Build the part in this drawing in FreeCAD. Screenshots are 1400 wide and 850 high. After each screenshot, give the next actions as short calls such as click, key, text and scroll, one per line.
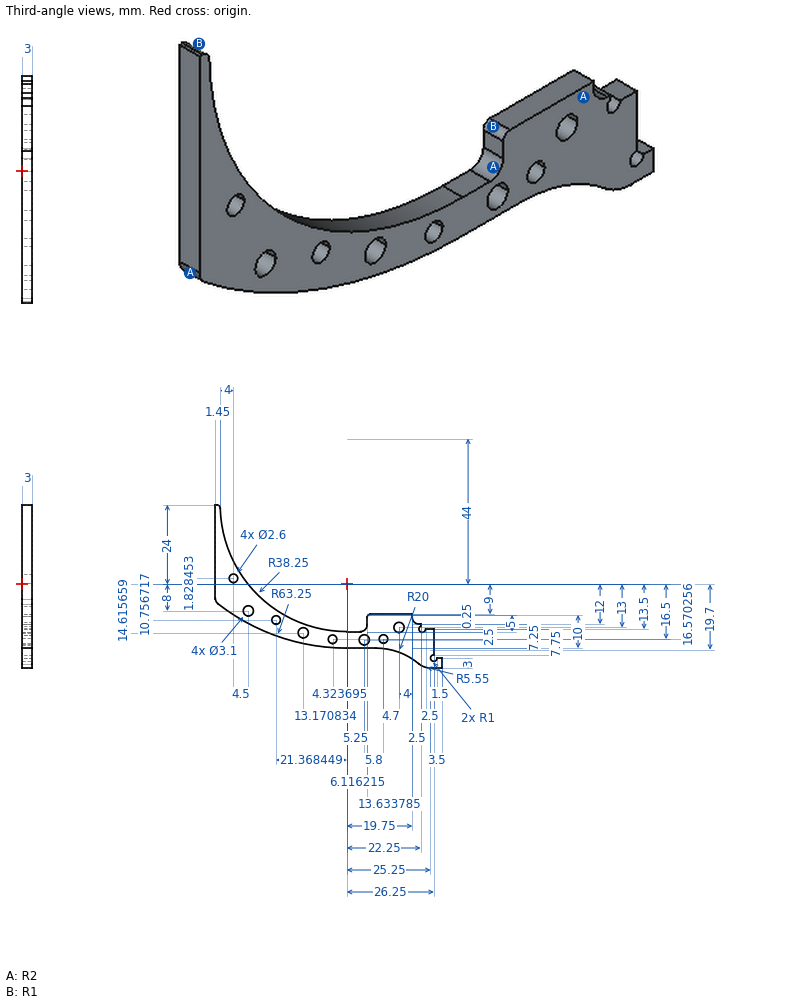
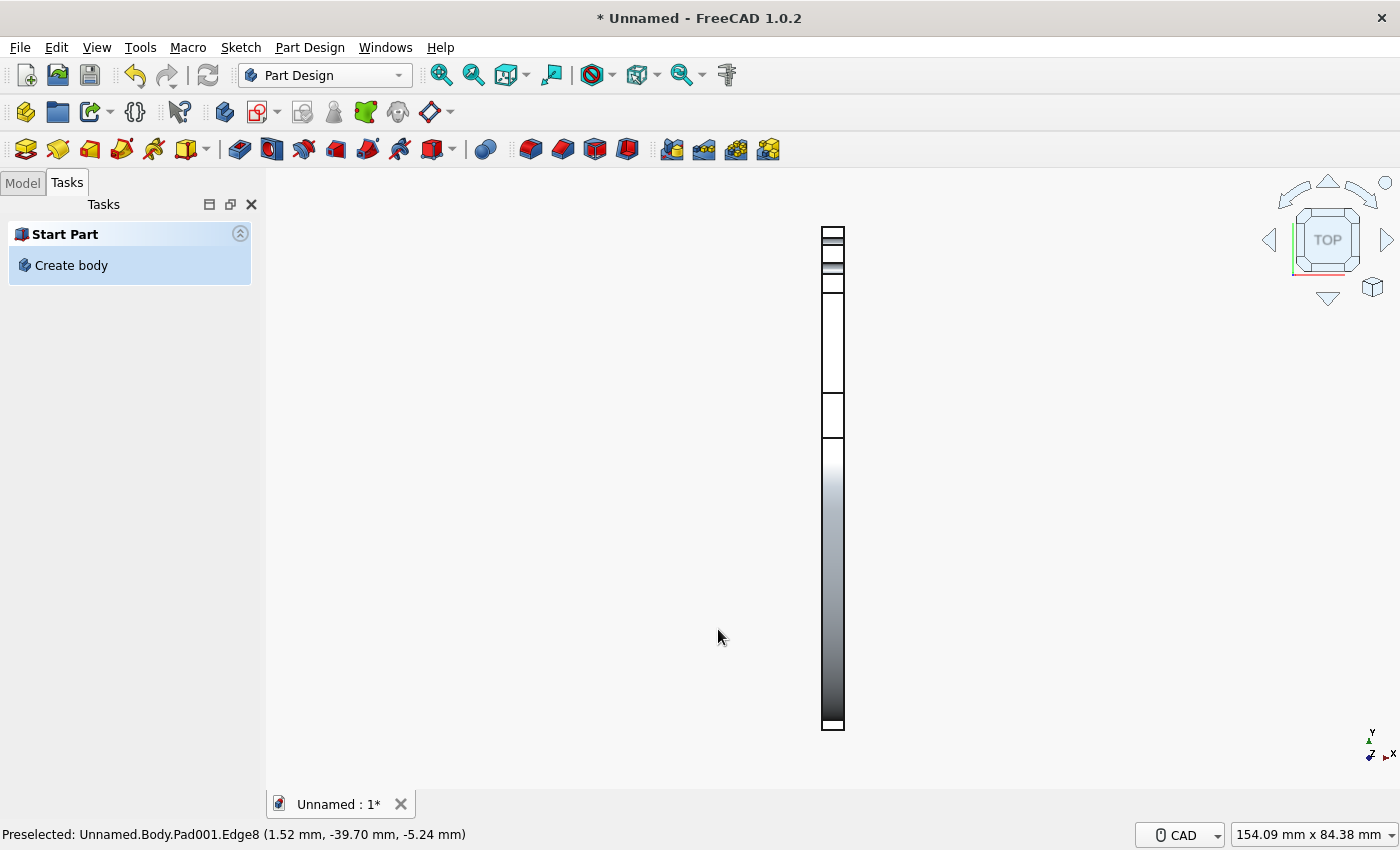
key(1)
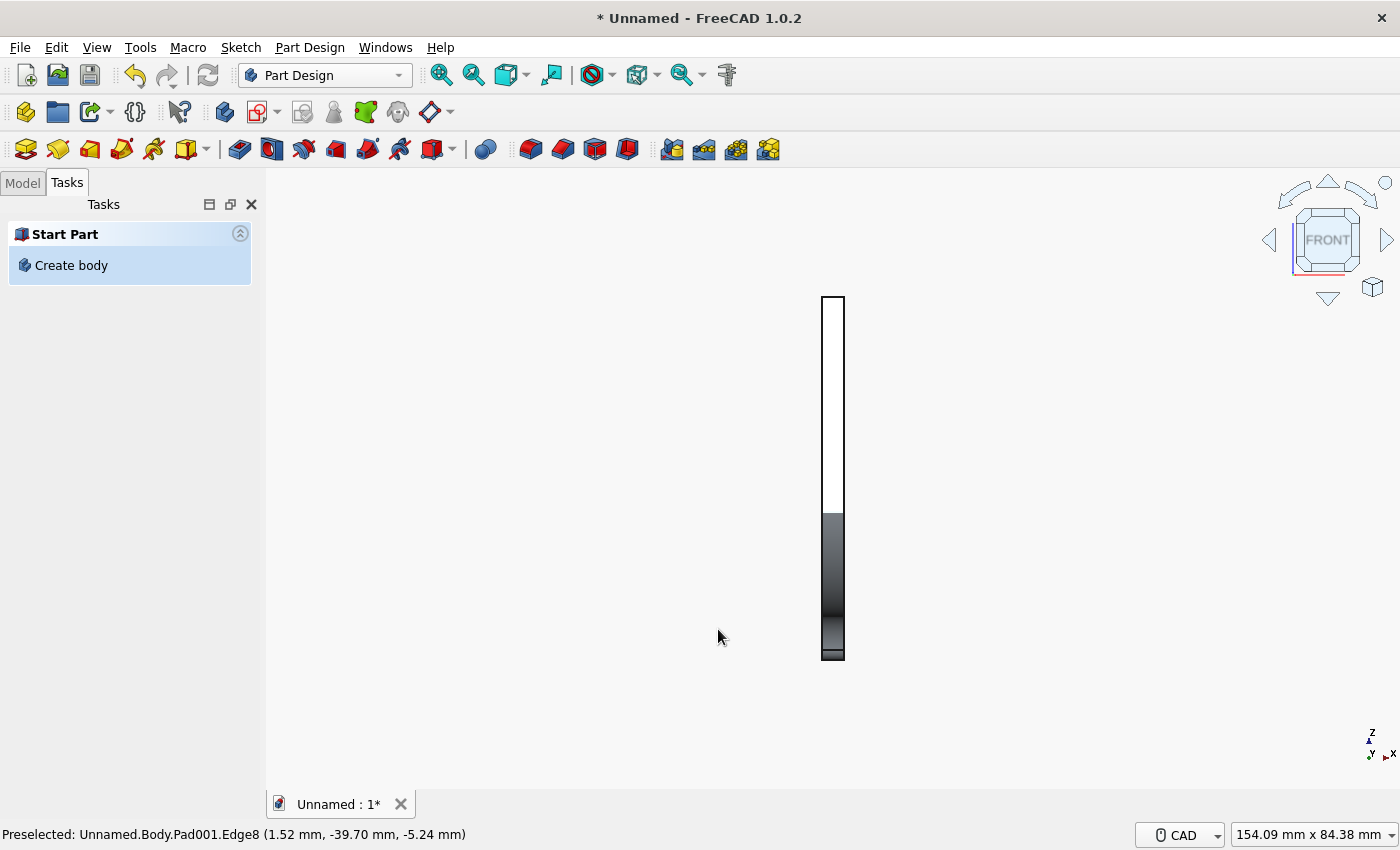
click(833, 511)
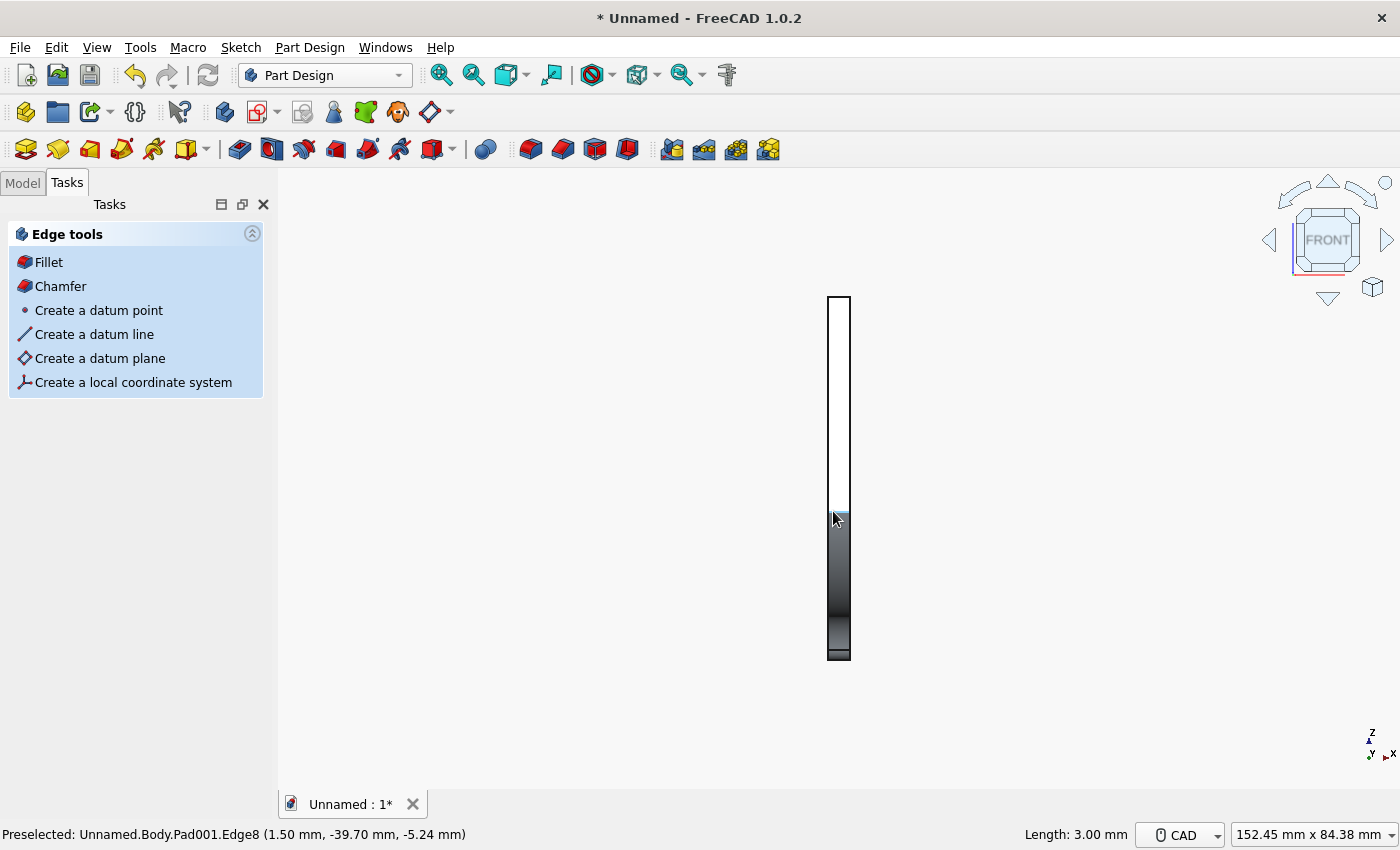
key(3)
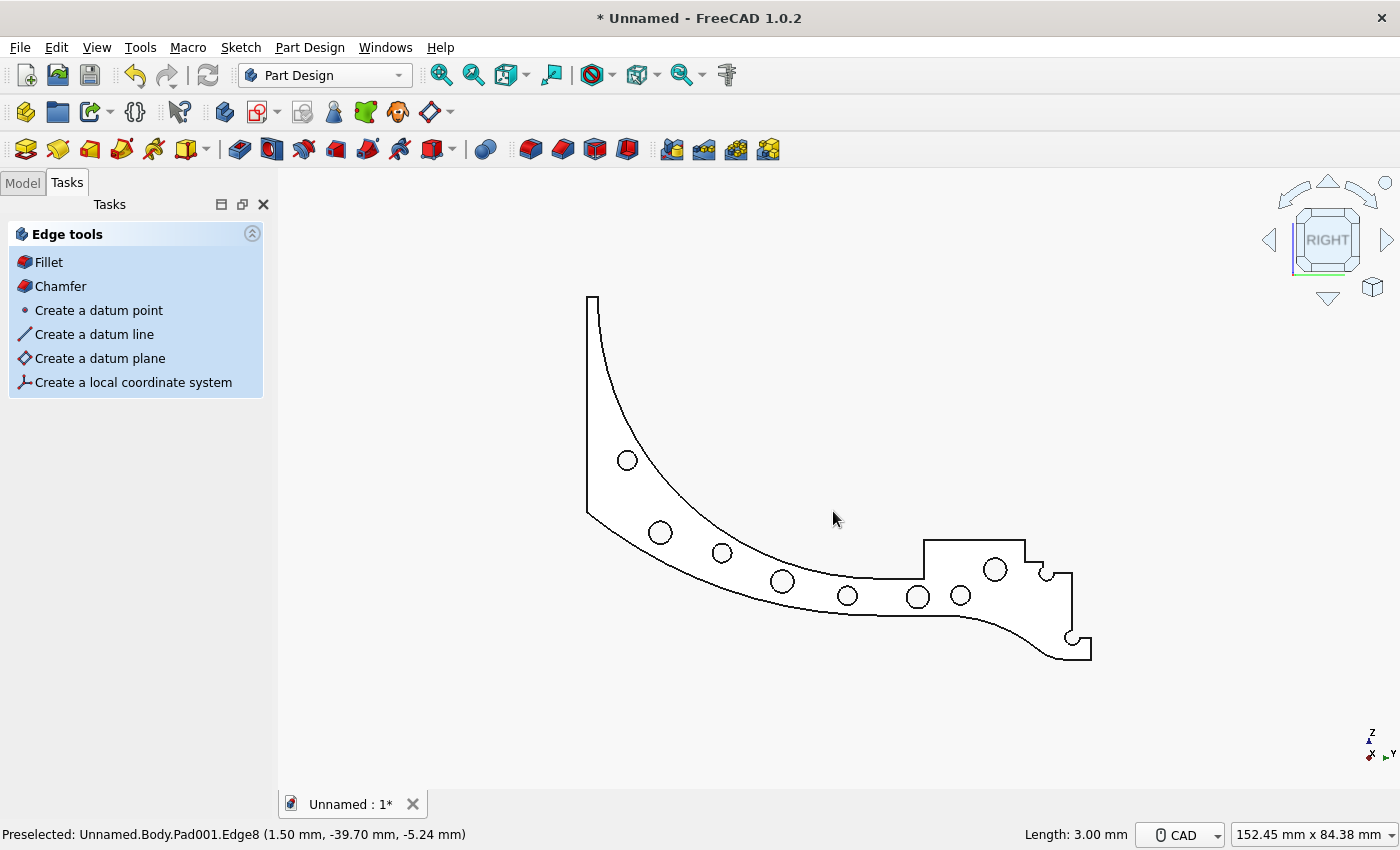
key(5)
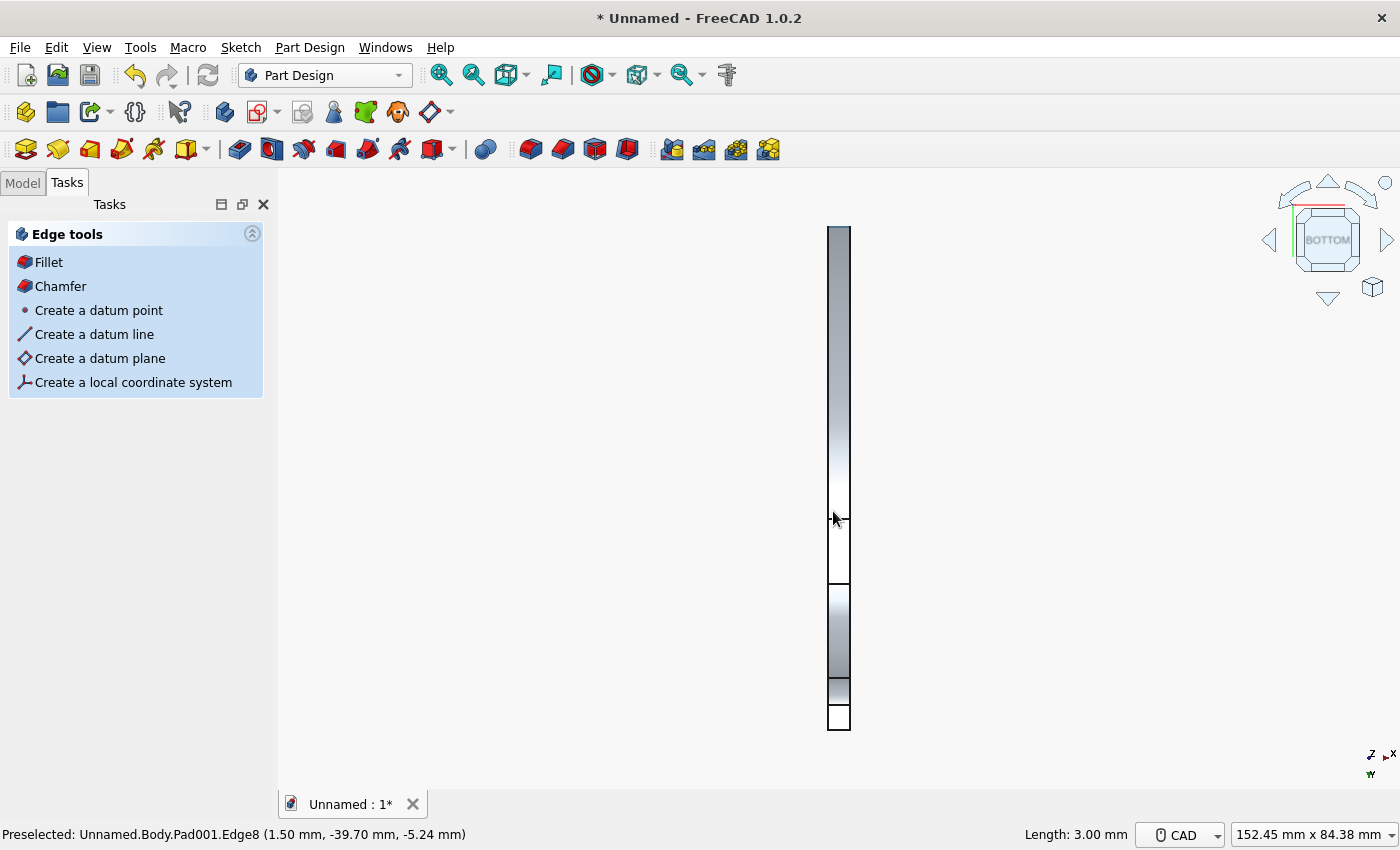
key(4)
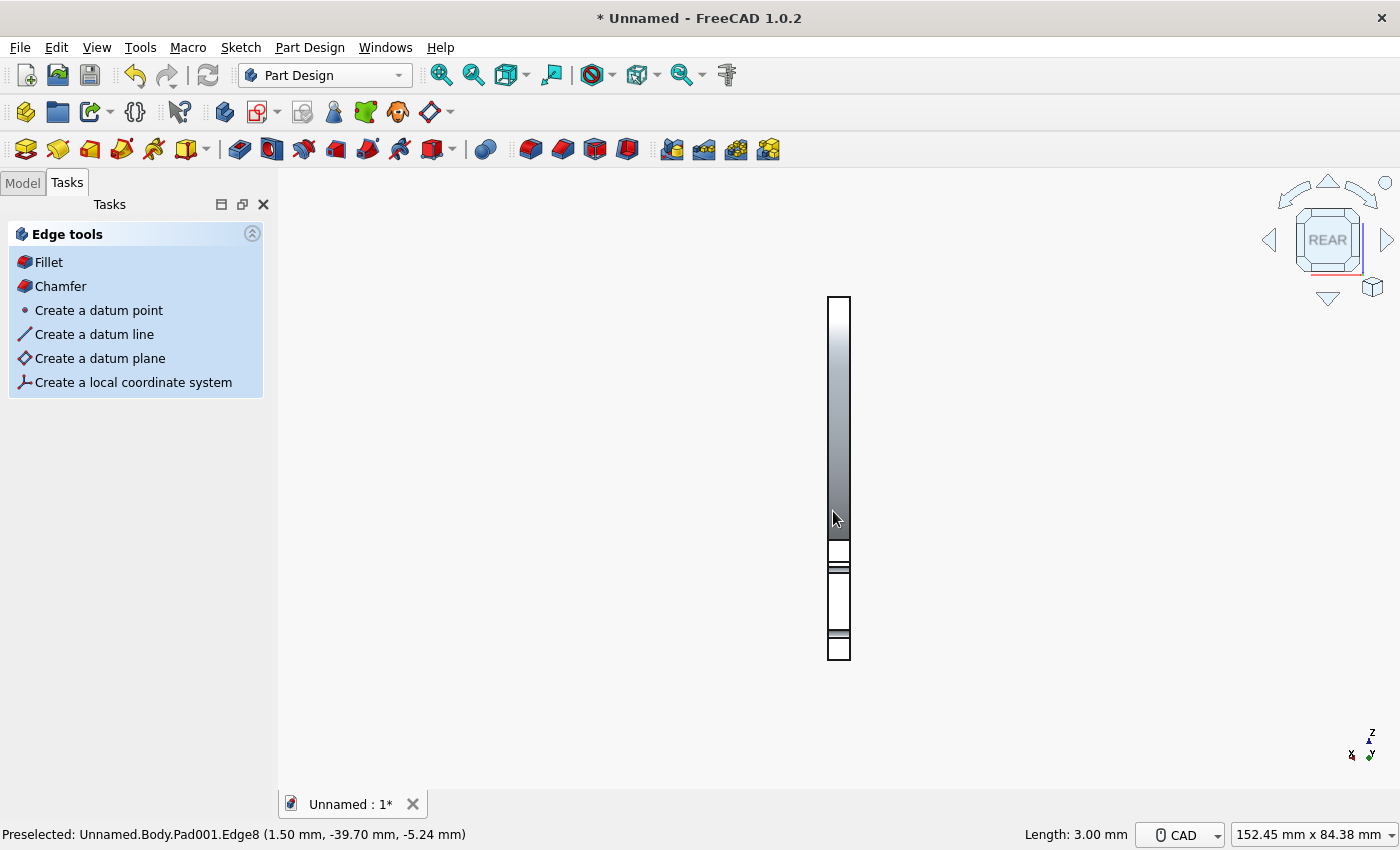
key(6)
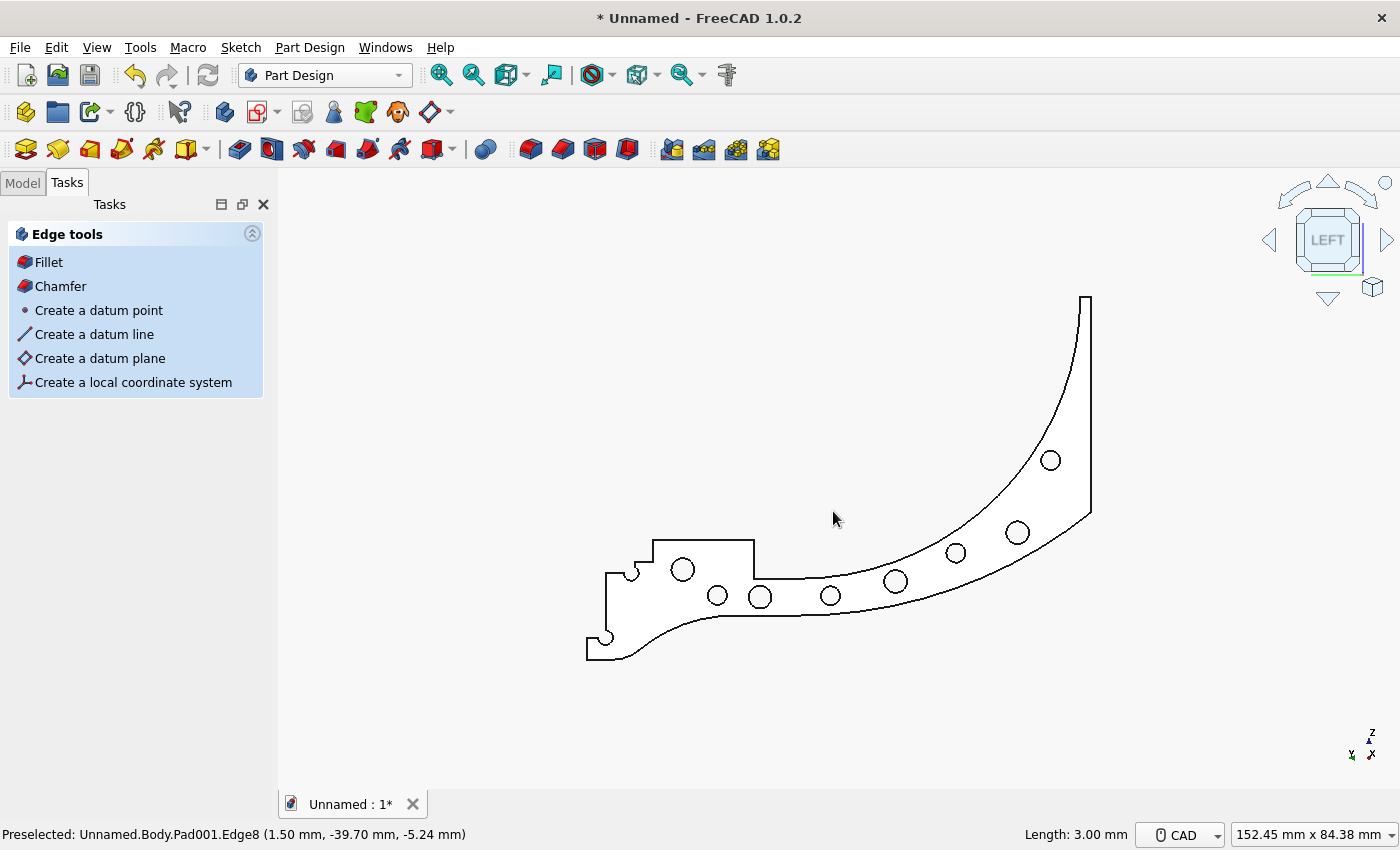
key(v)
key(3)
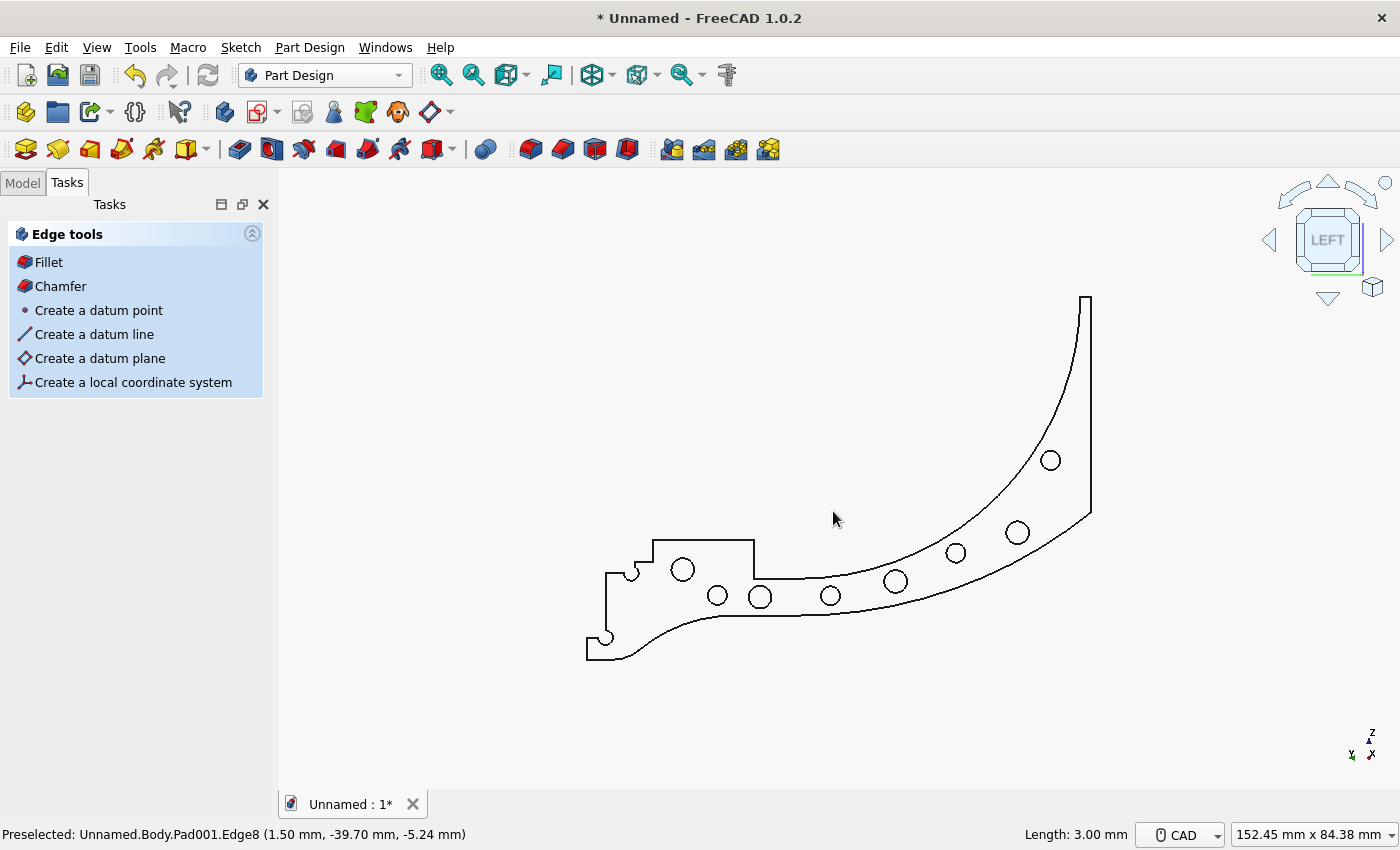
key(0)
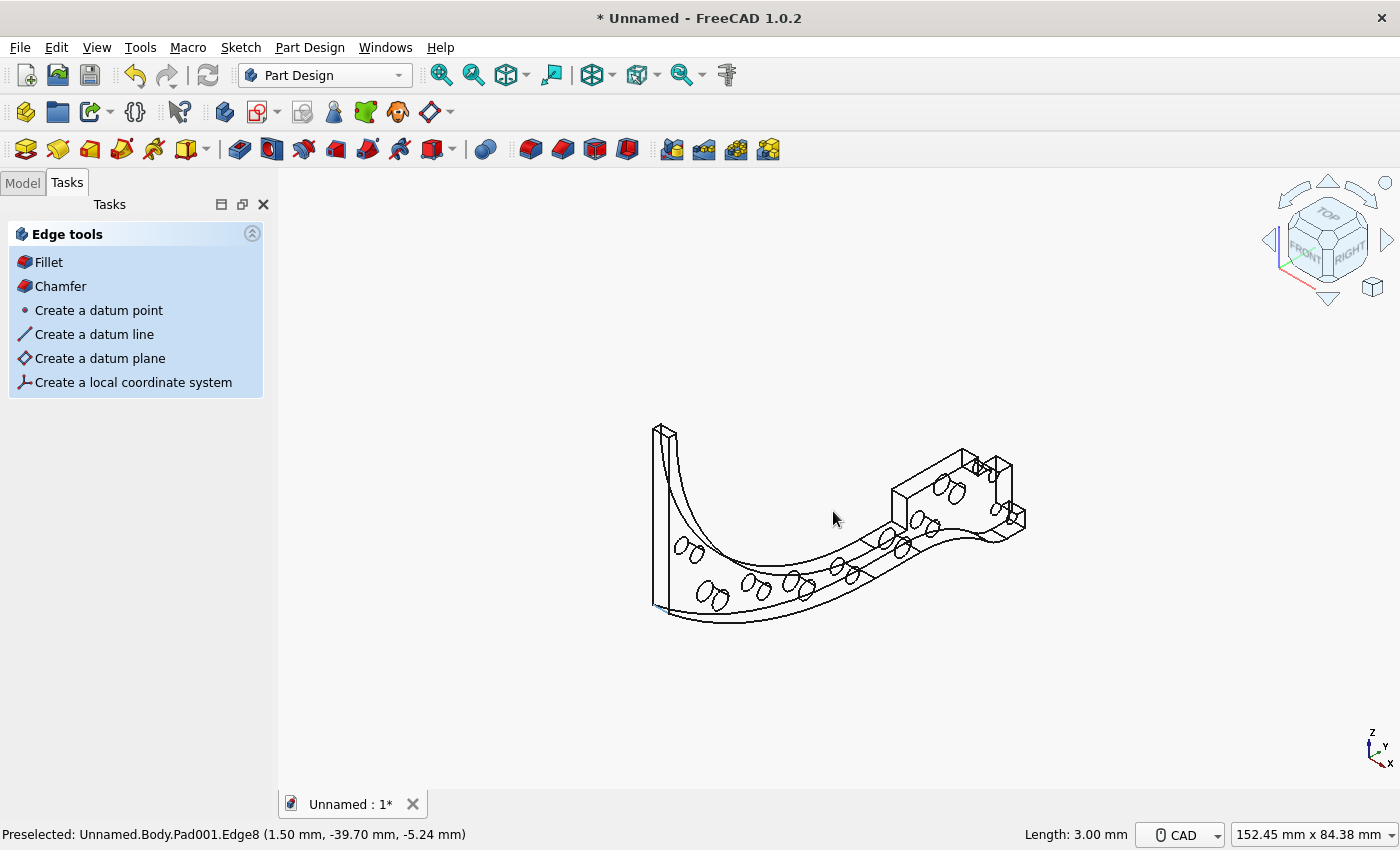
click(899, 525, ctrl)